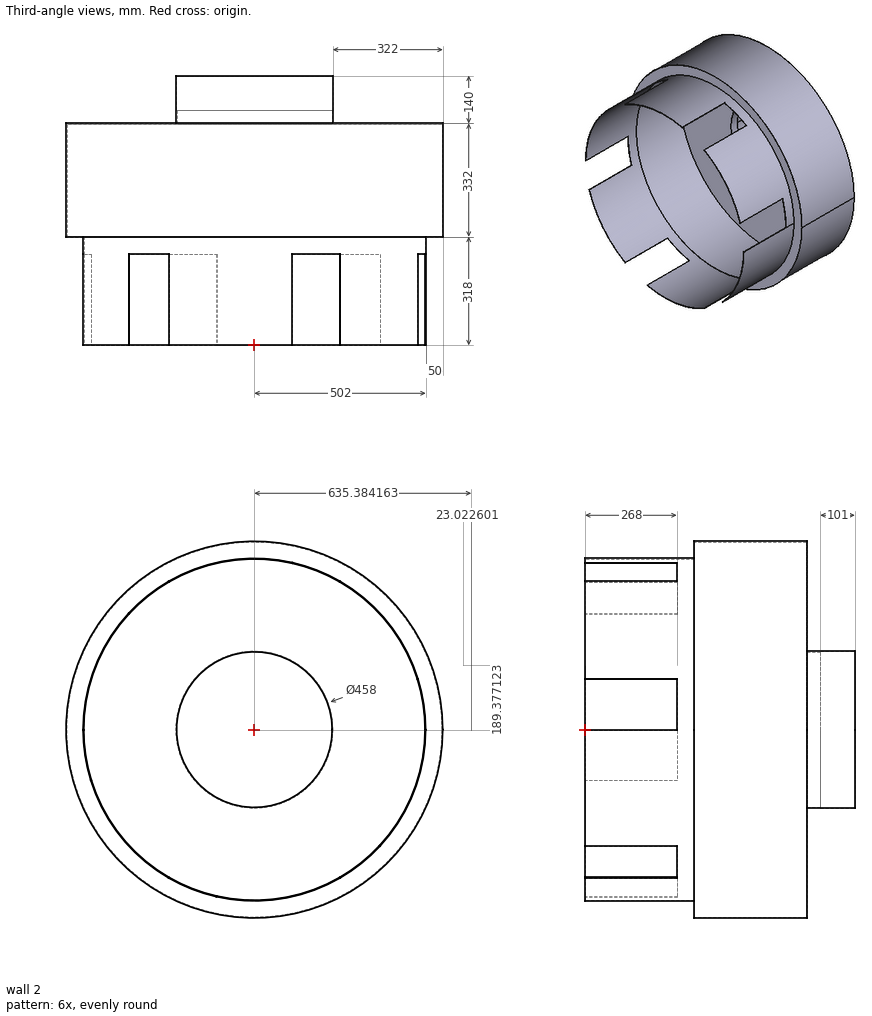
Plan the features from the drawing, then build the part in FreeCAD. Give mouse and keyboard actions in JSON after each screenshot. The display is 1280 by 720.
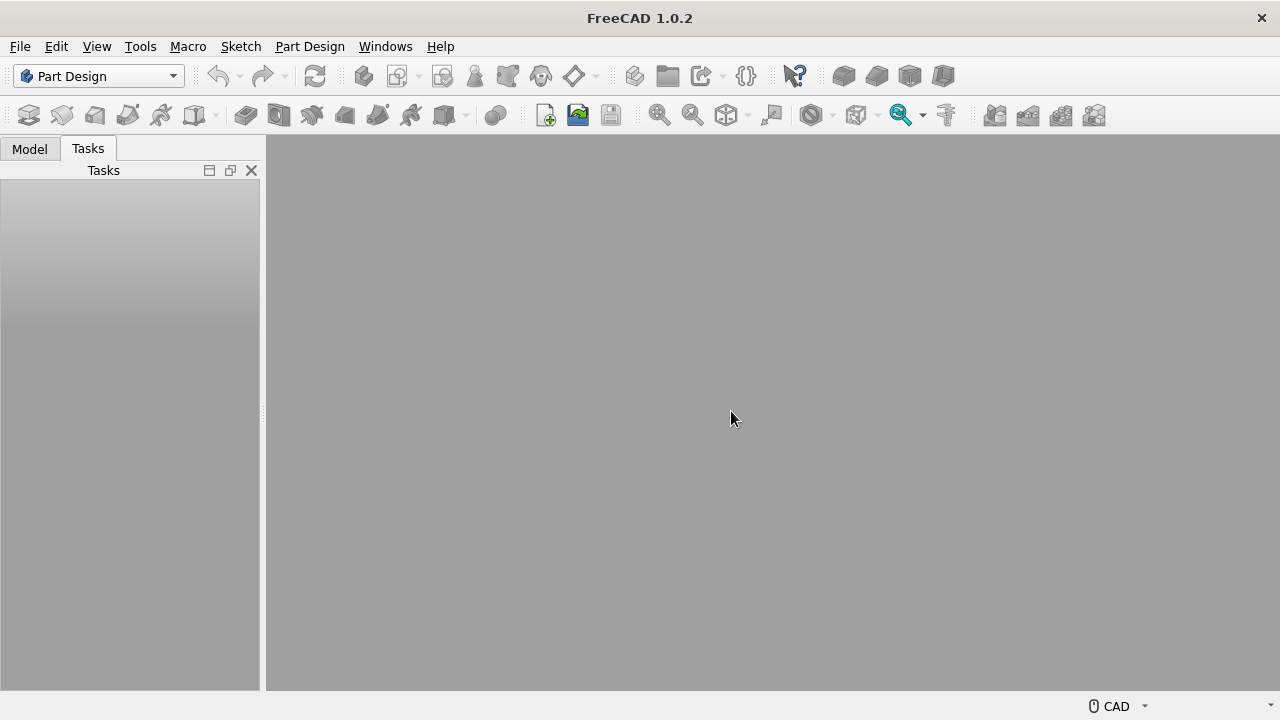
{"action": "key", "text": "ctrl+n"}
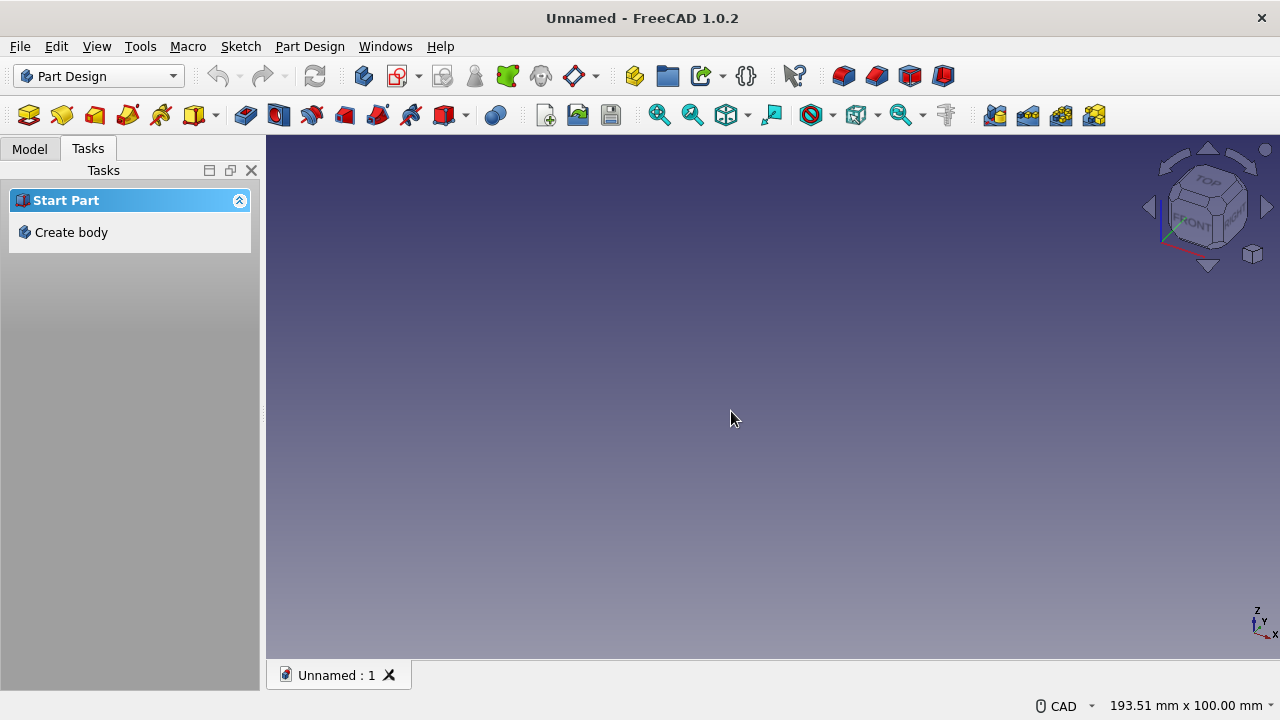
{"action": "left_click", "coordinate": [396, 76]}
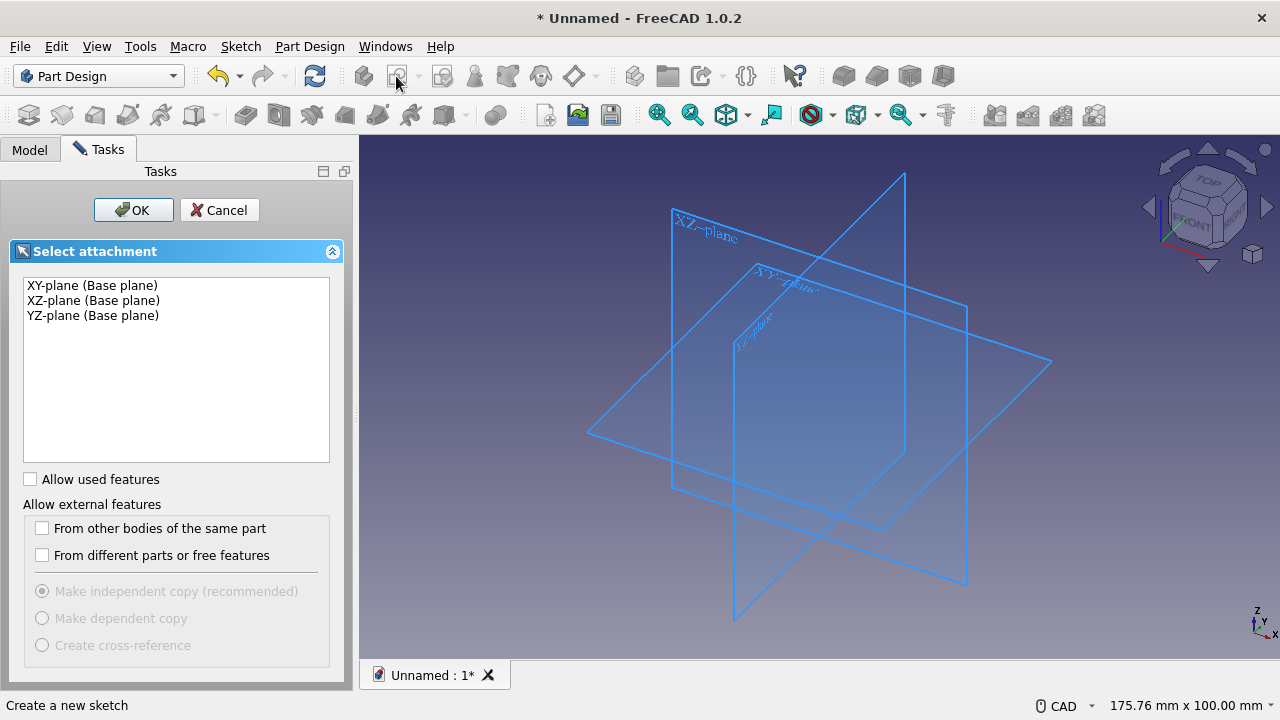
{"action": "left_click", "coordinate": [84, 286]}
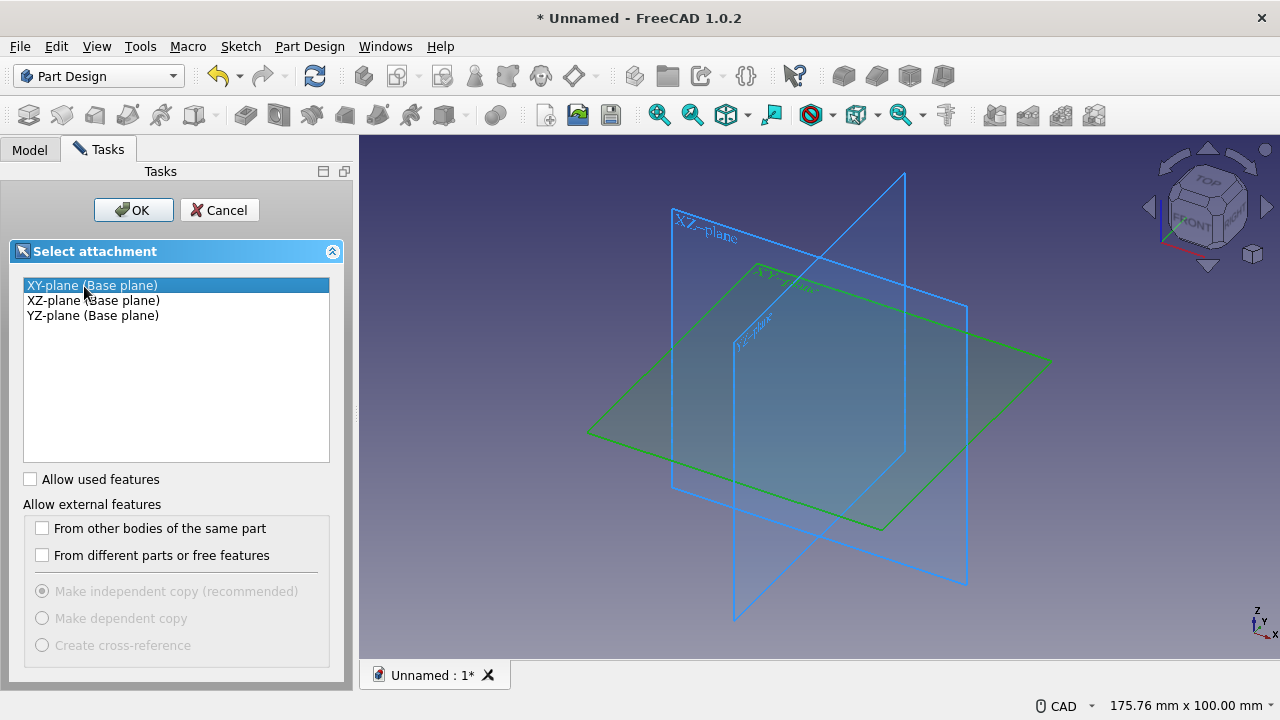
{"action": "left_click", "coordinate": [134, 210]}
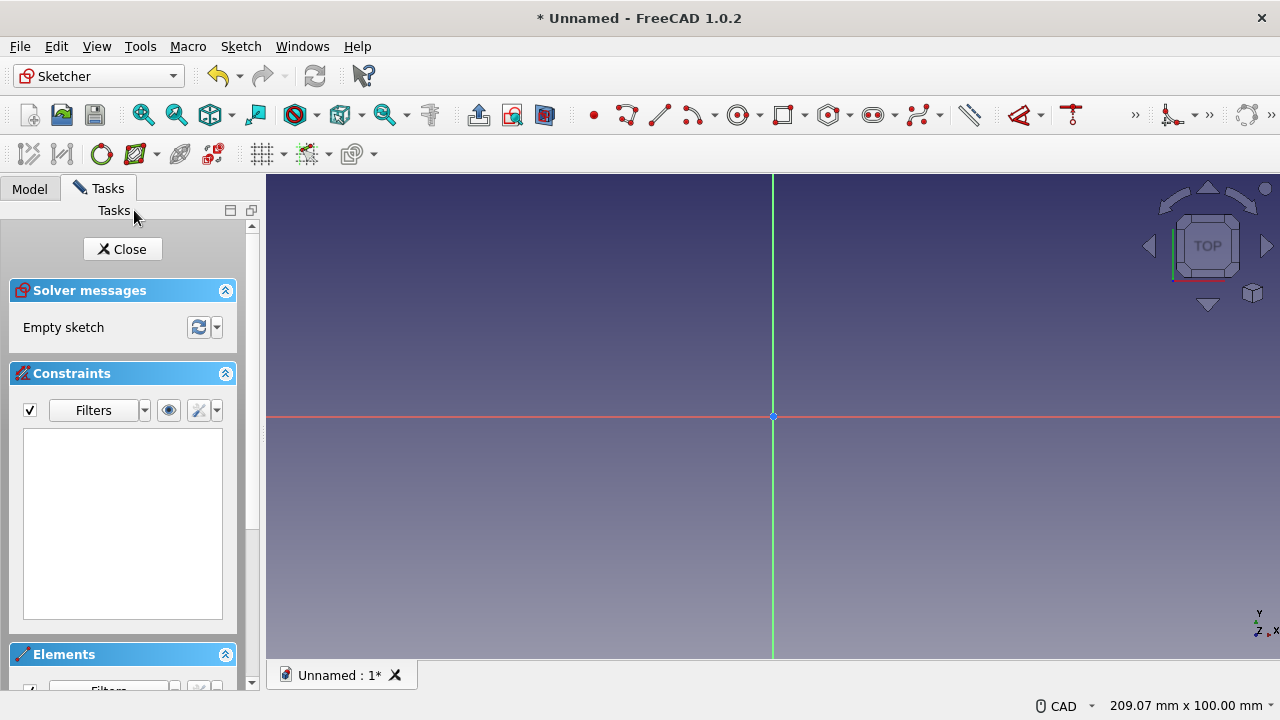
{"action": "scroll", "coordinate": [592, 570], "scroll_direction": "down", "scroll_amount": 13}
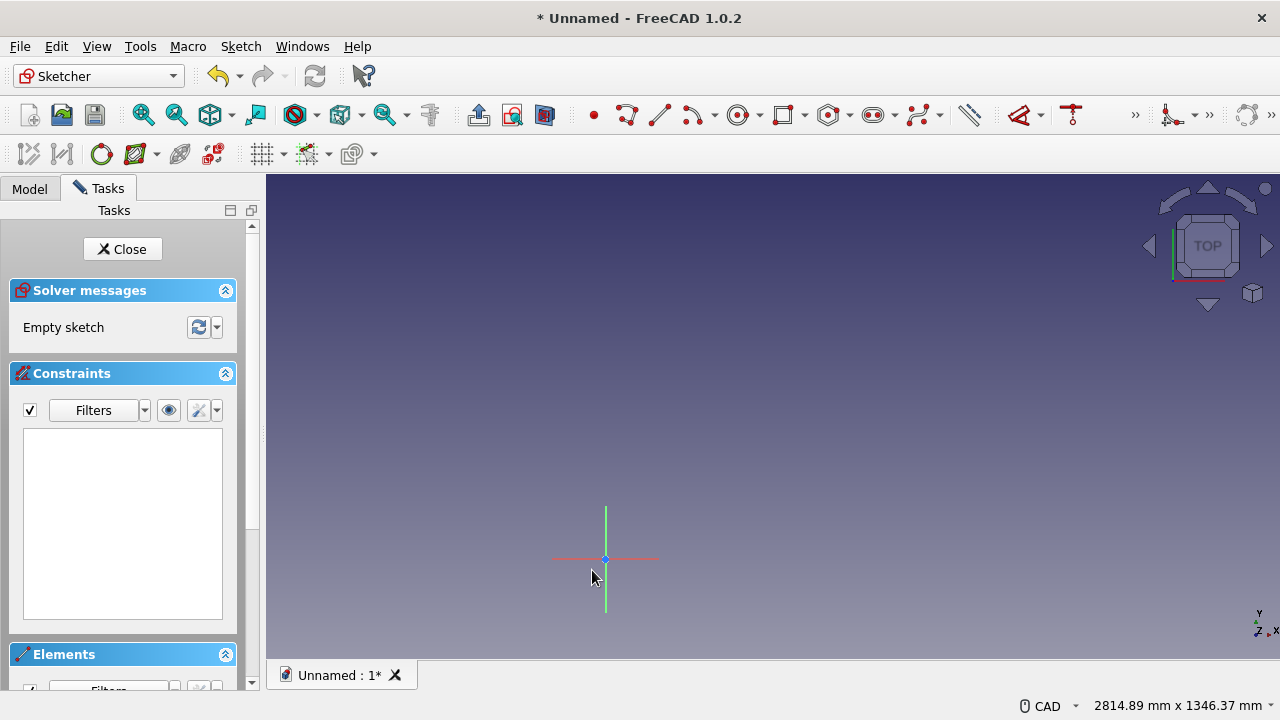
{"action": "left_click", "coordinate": [627, 116]}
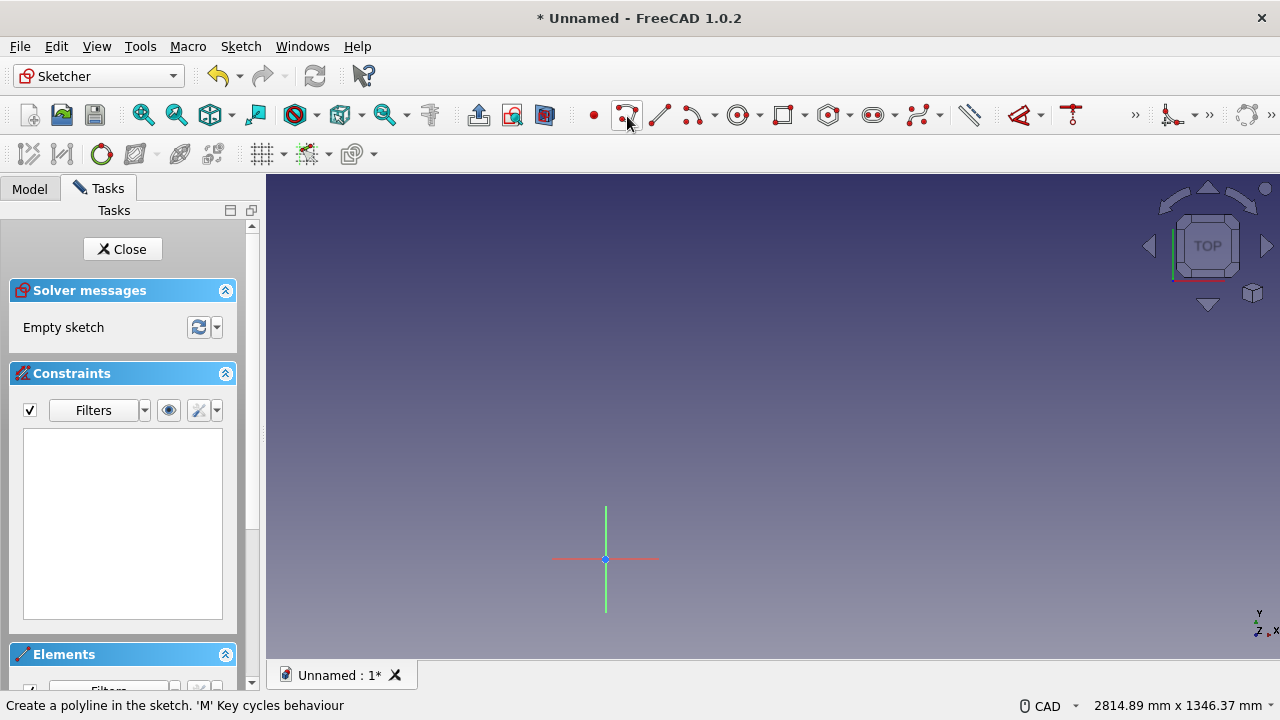
{"action": "left_click", "coordinate": [606, 559]}
{"action": "left_click", "coordinate": [787, 550]}
{"action": "left_click", "coordinate": [787, 445]}
{"action": "left_click", "coordinate": [805, 445]}
{"action": "left_click", "coordinate": [805, 325]}
{"action": "left_click", "coordinate": [689, 325]}
{"action": "left_click", "coordinate": [689, 275]}
{"action": "left_click", "coordinate": [615, 275]}
{"action": "left_click", "coordinate": [606, 559]}
{"action": "key", "text": "Escape"}
{"action": "key", "text": "Escape"}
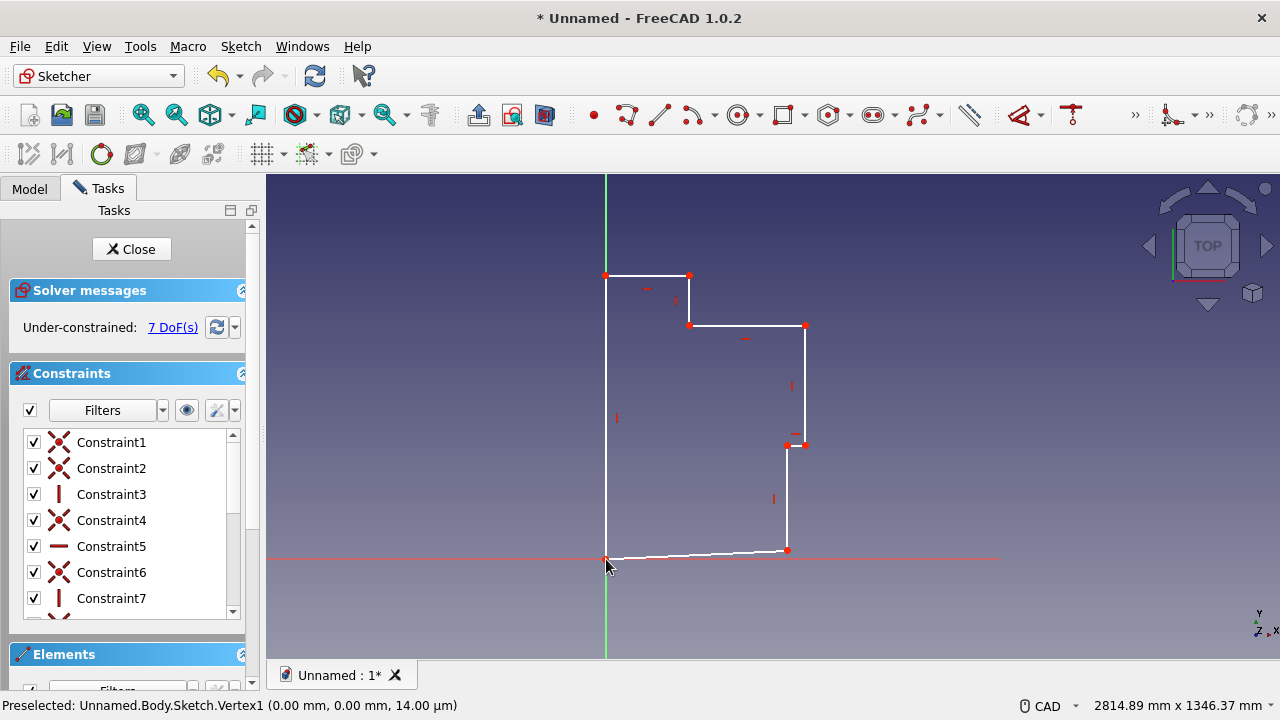
{"action": "left_click", "coordinate": [660, 557]}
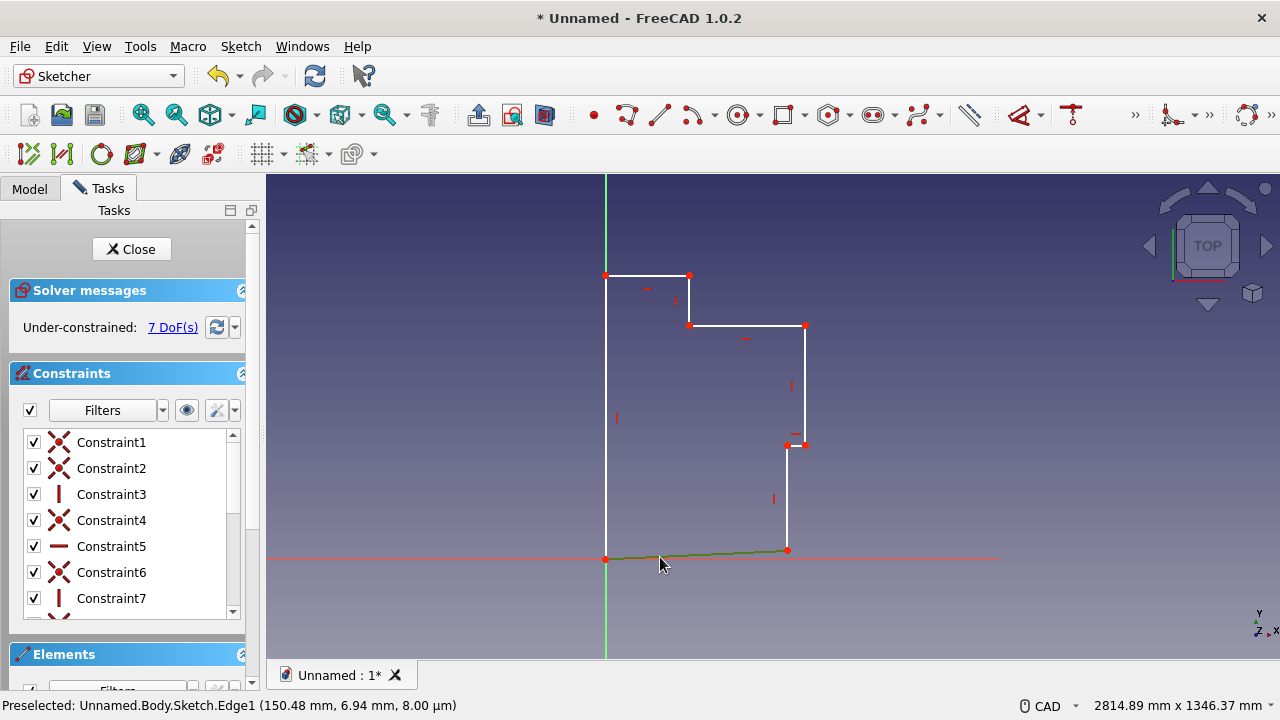
{"action": "key", "text": "h"}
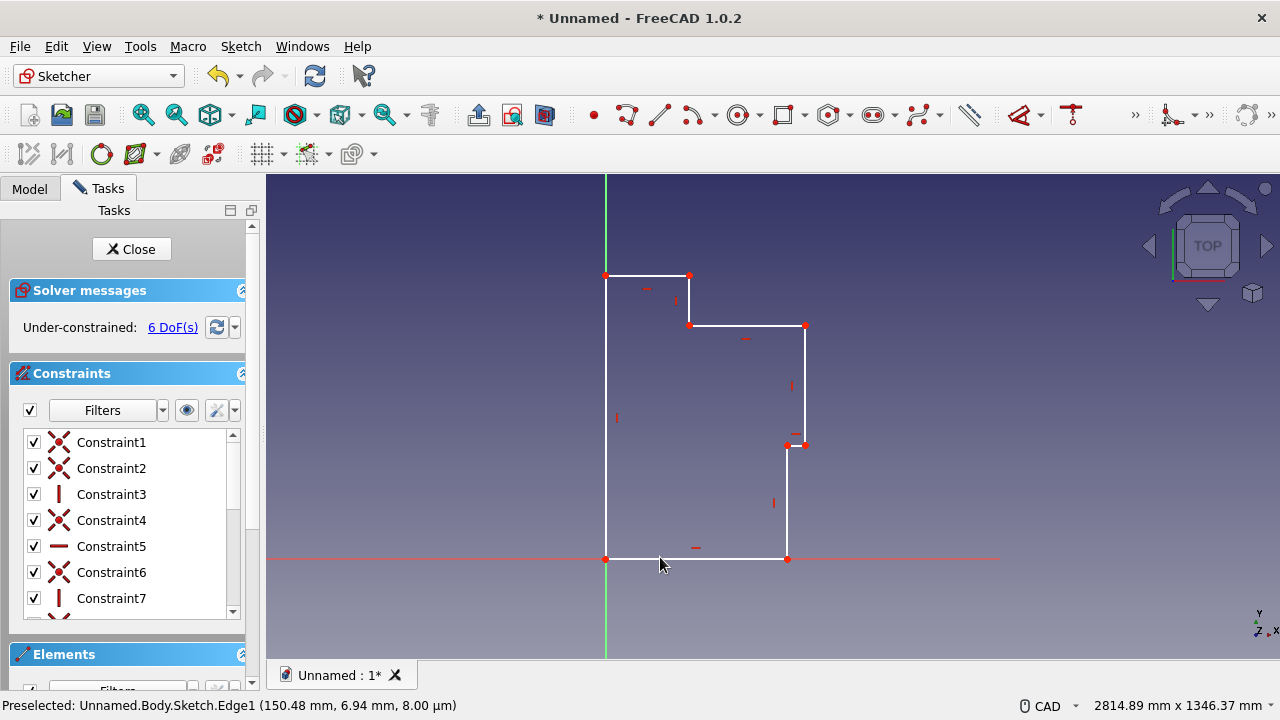
{"action": "left_click", "coordinate": [1018, 116]}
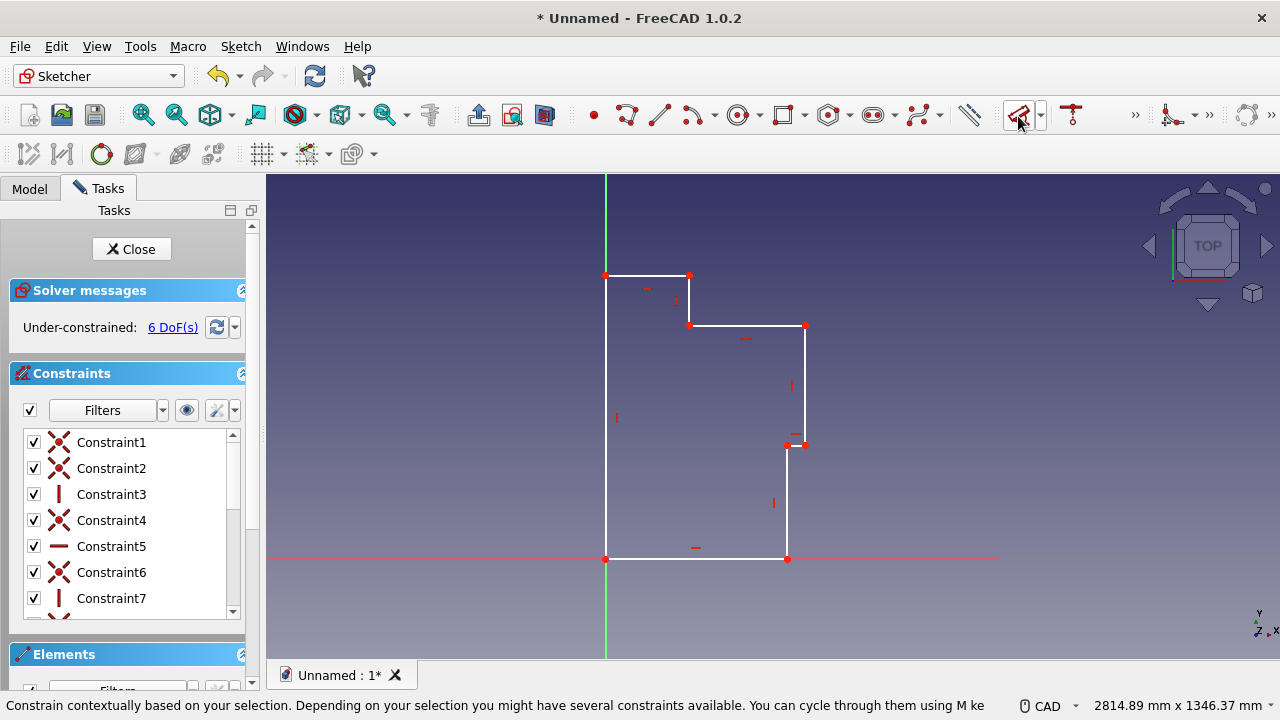
{"action": "scroll", "coordinate": [796, 446], "scroll_direction": "up", "scroll_amount": 4}